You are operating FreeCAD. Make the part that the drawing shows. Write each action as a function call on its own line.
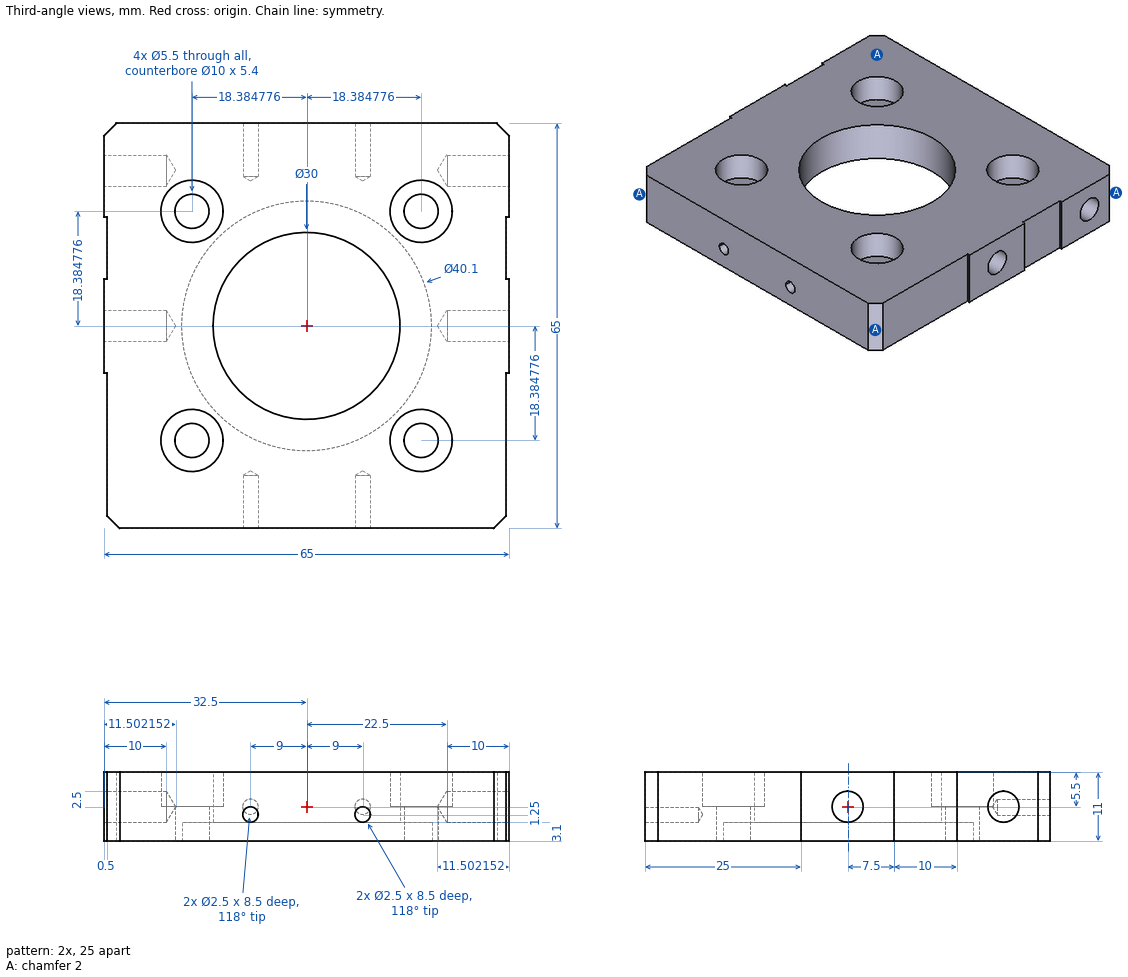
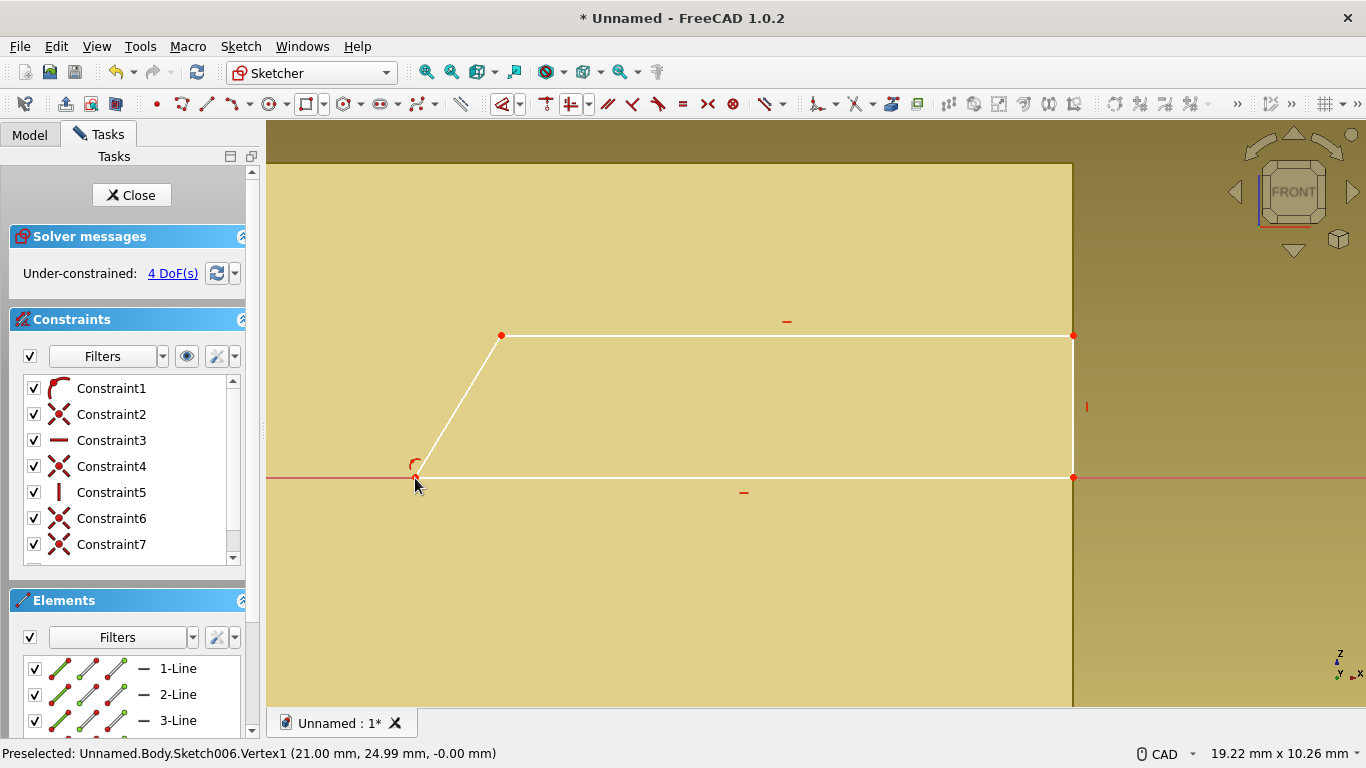
click(673, 336)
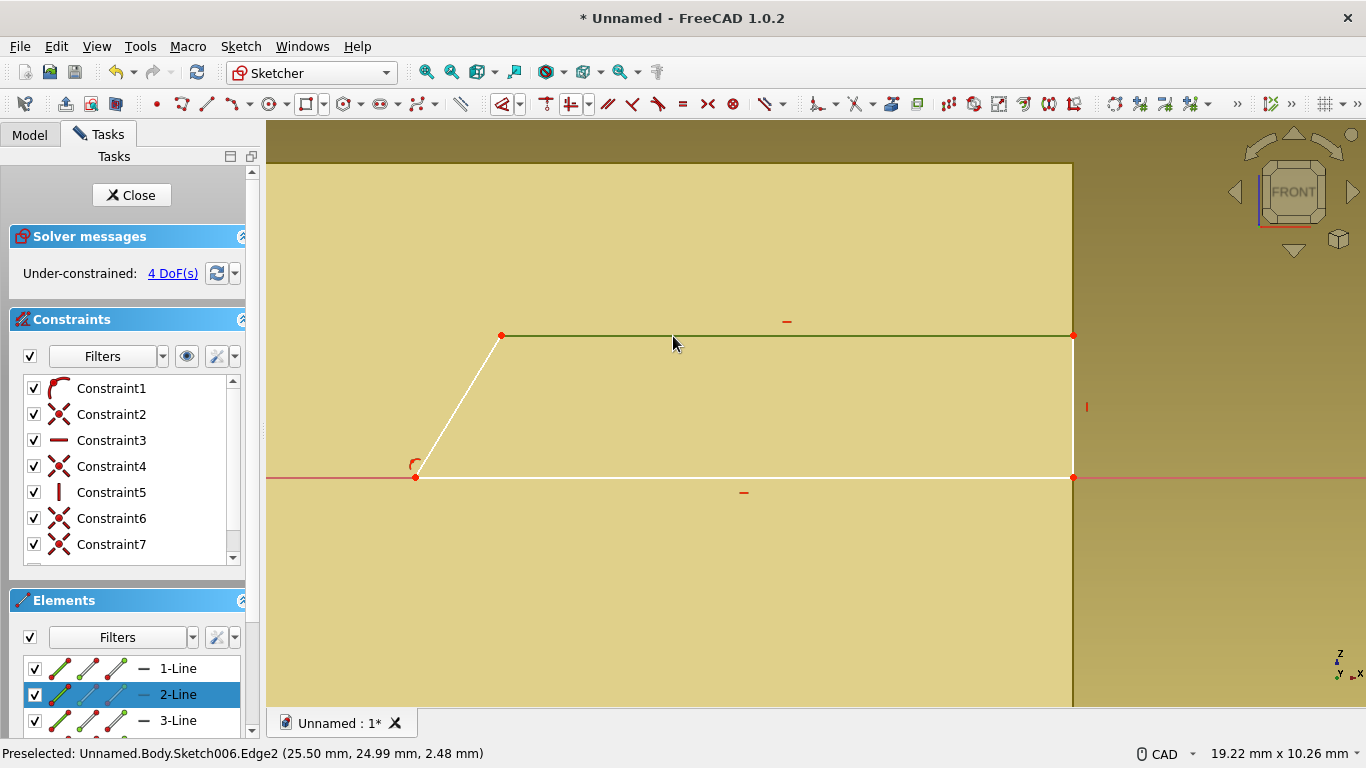
click(520, 104)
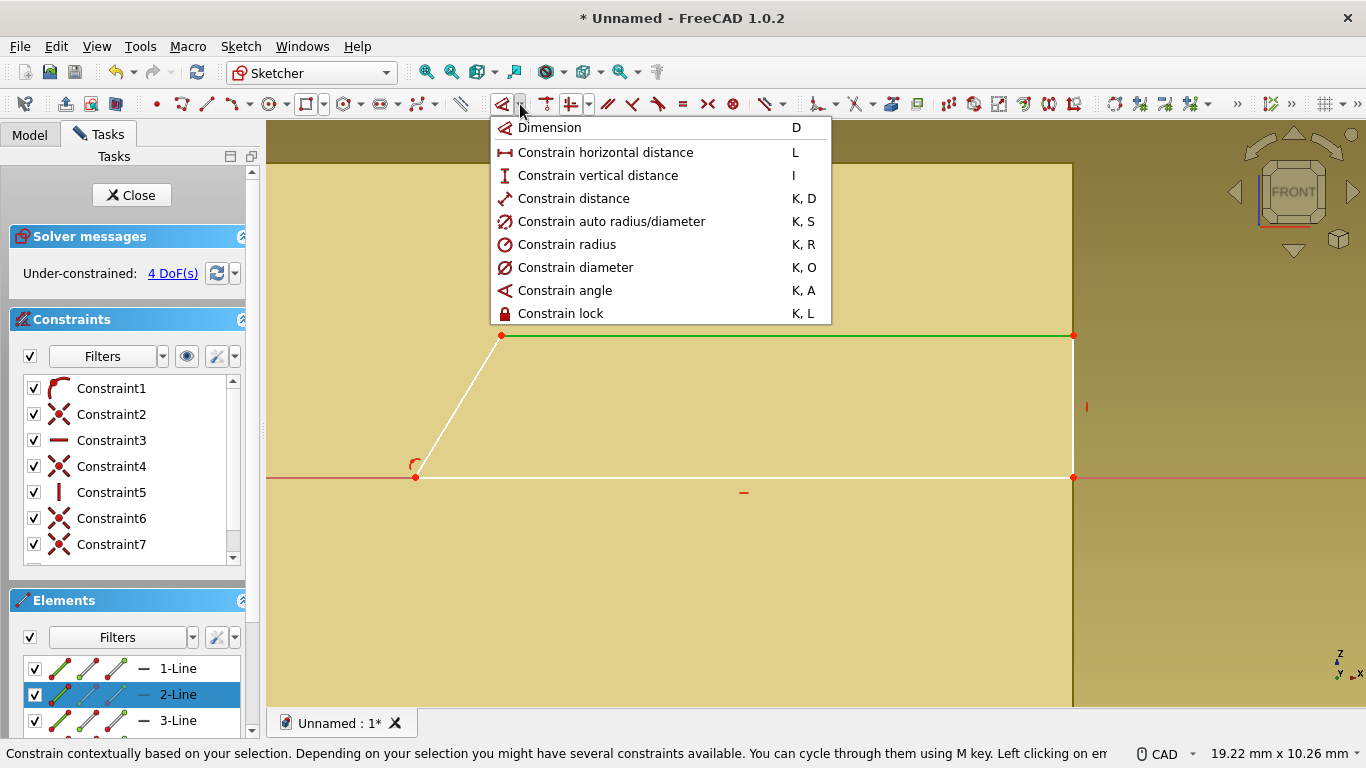
click(661, 152)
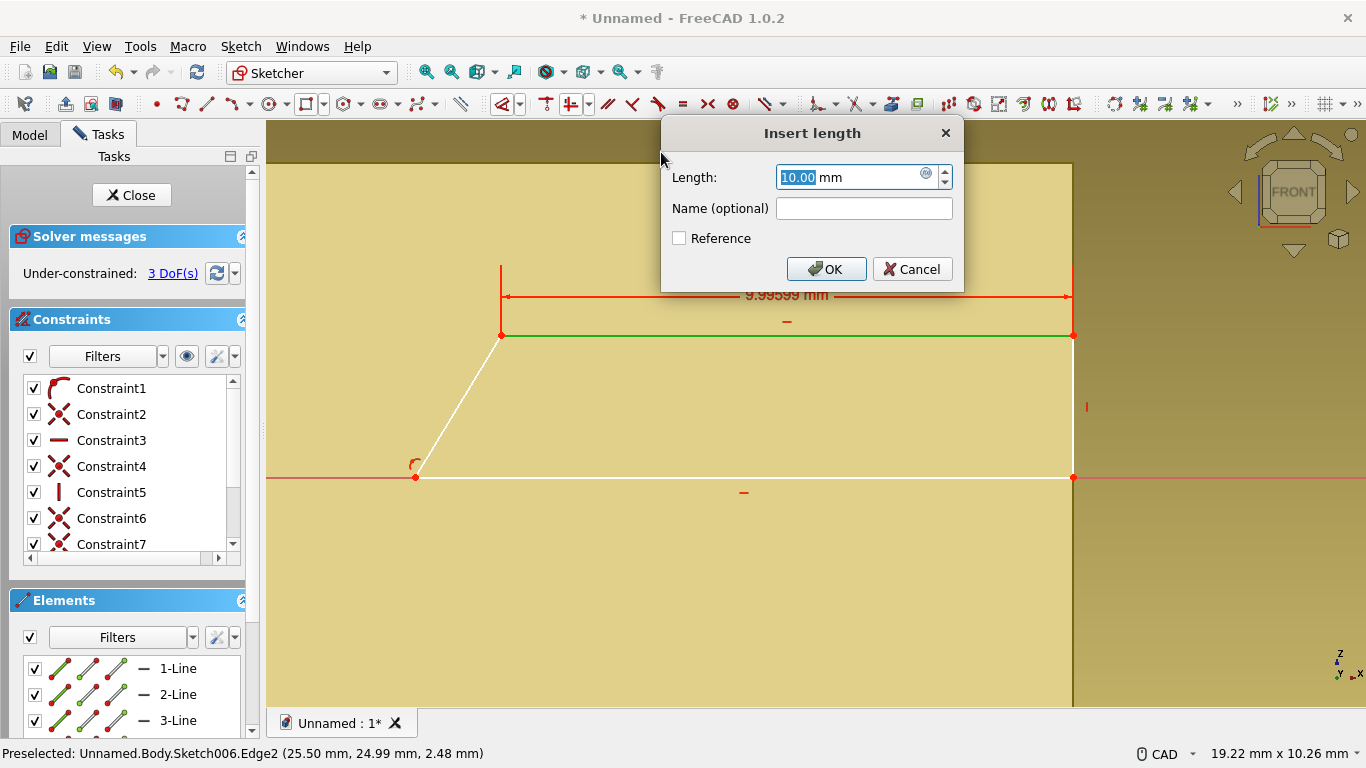
text(10)
key(Return)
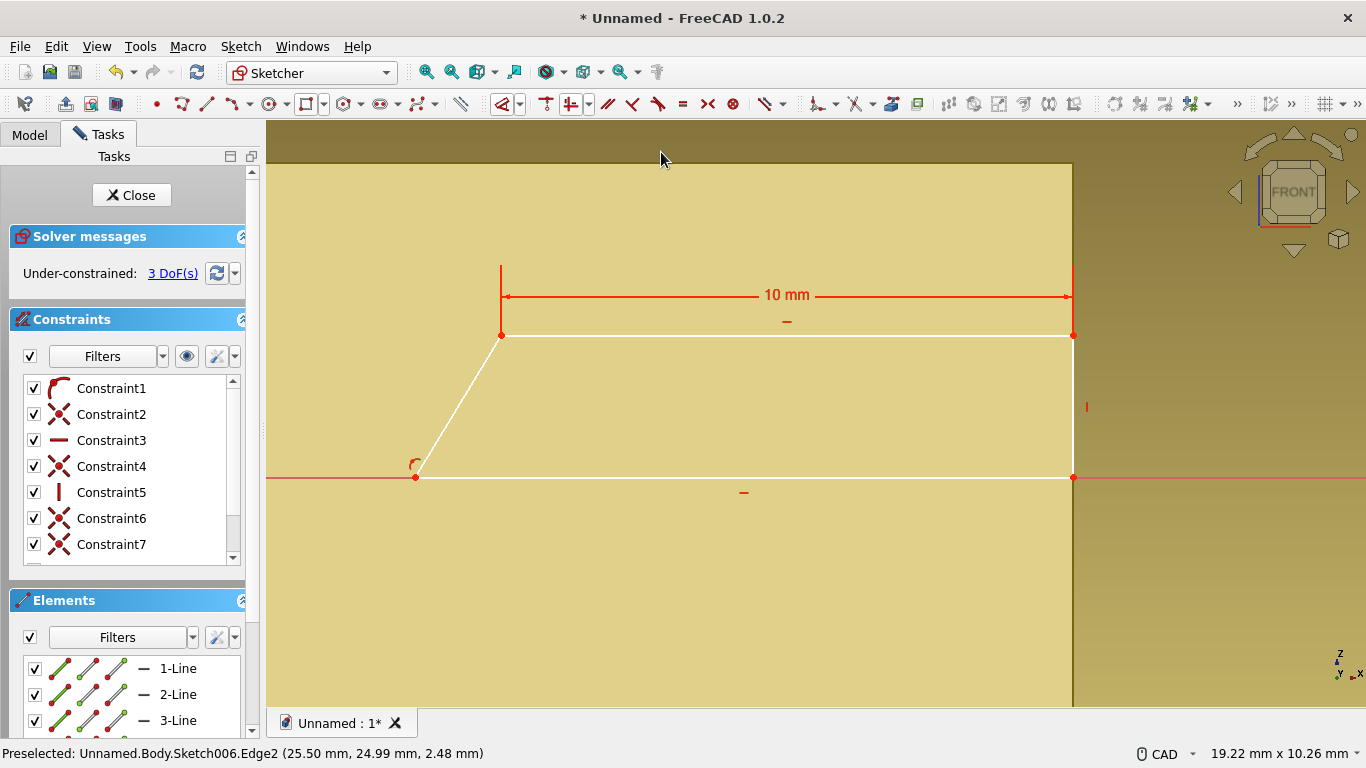
click(1073, 379)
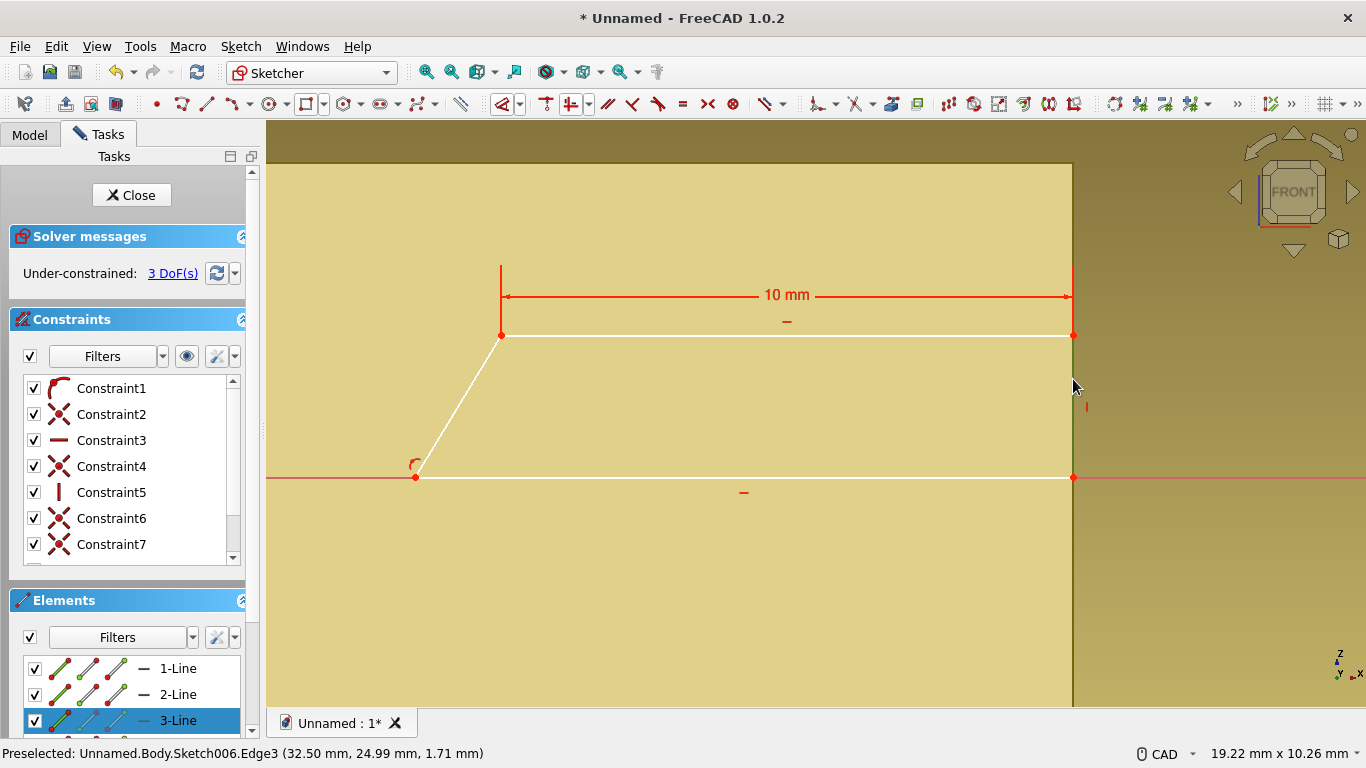
key(i)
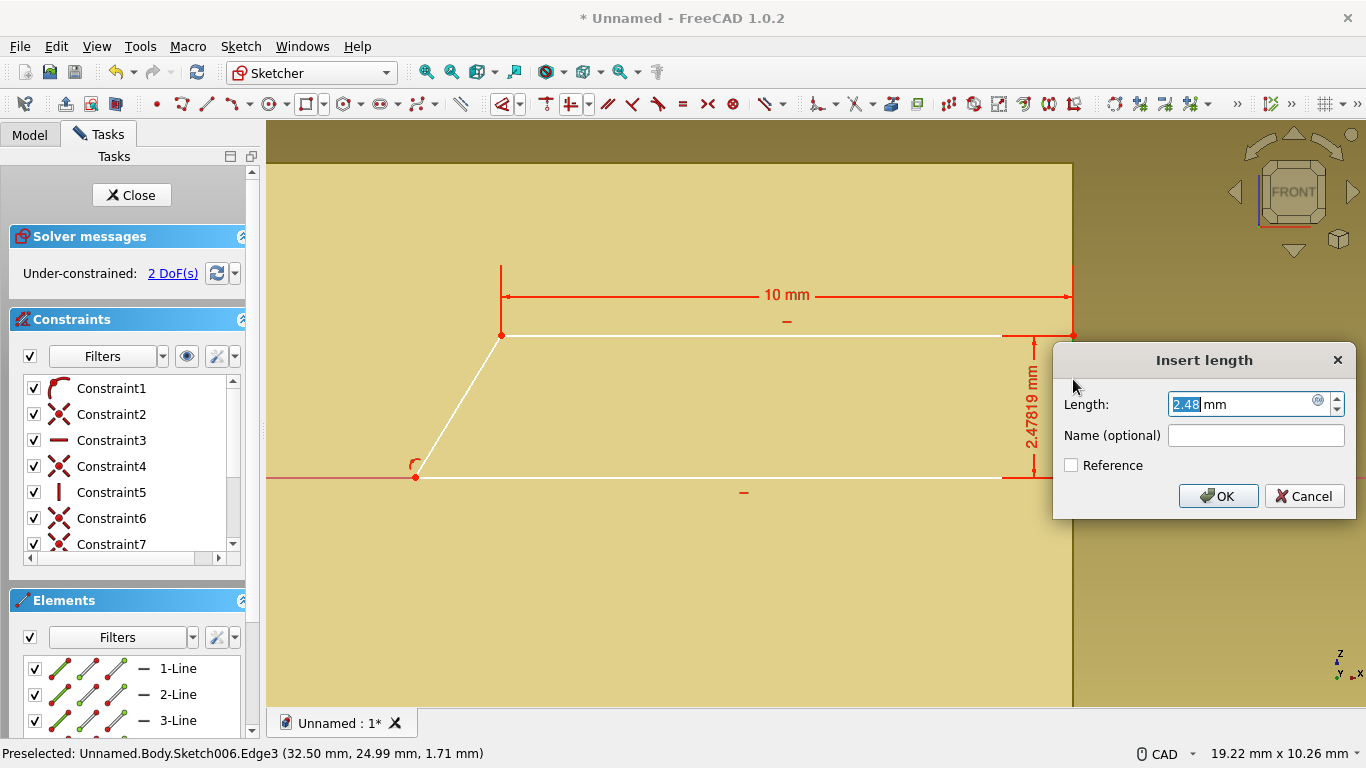
text(2.5)
key(Return)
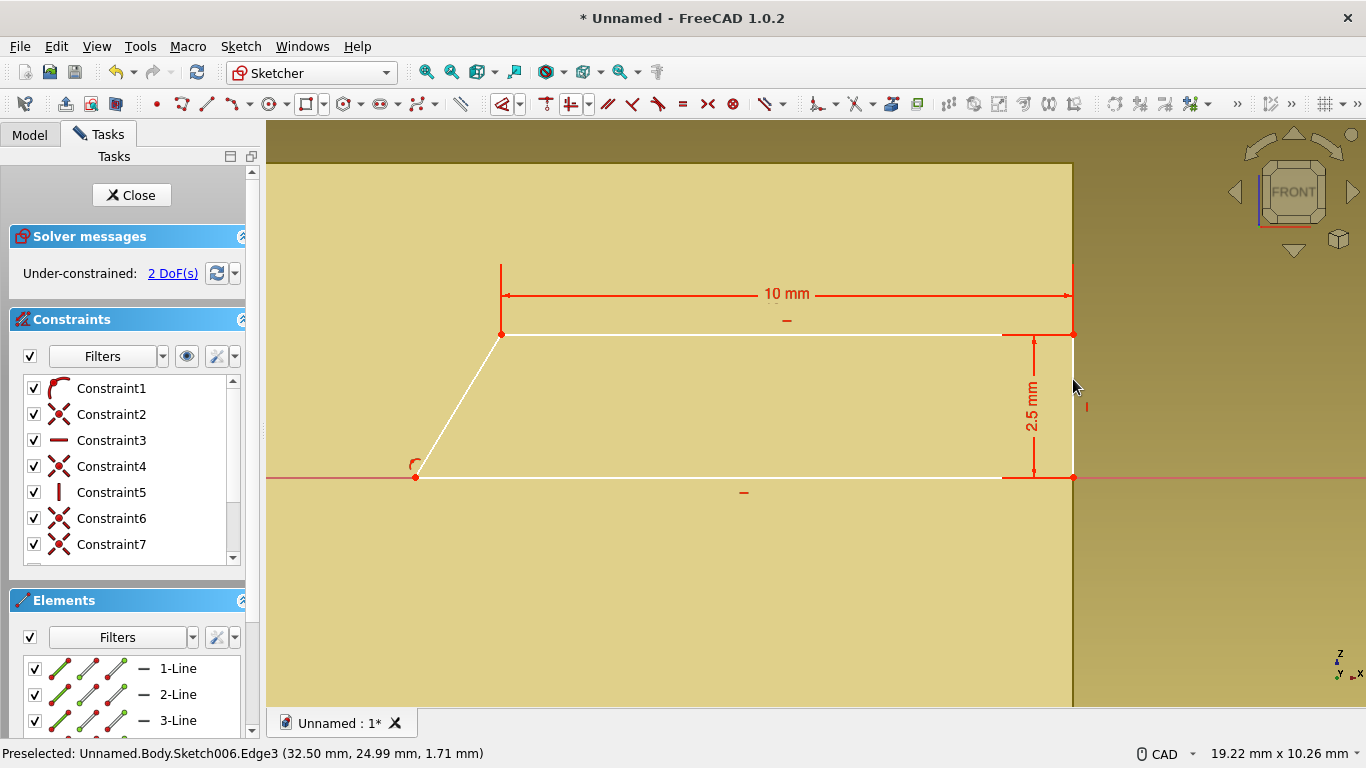
click(501, 335)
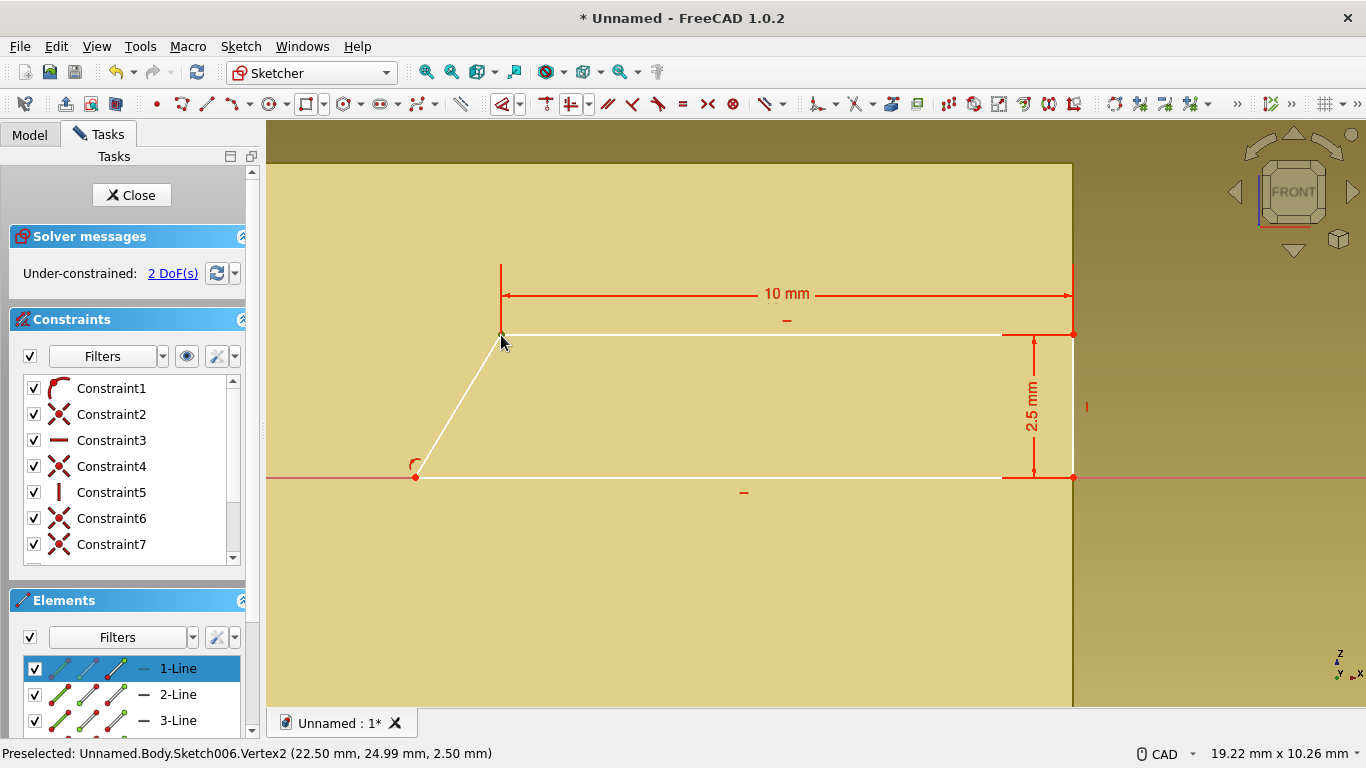
click(520, 104)